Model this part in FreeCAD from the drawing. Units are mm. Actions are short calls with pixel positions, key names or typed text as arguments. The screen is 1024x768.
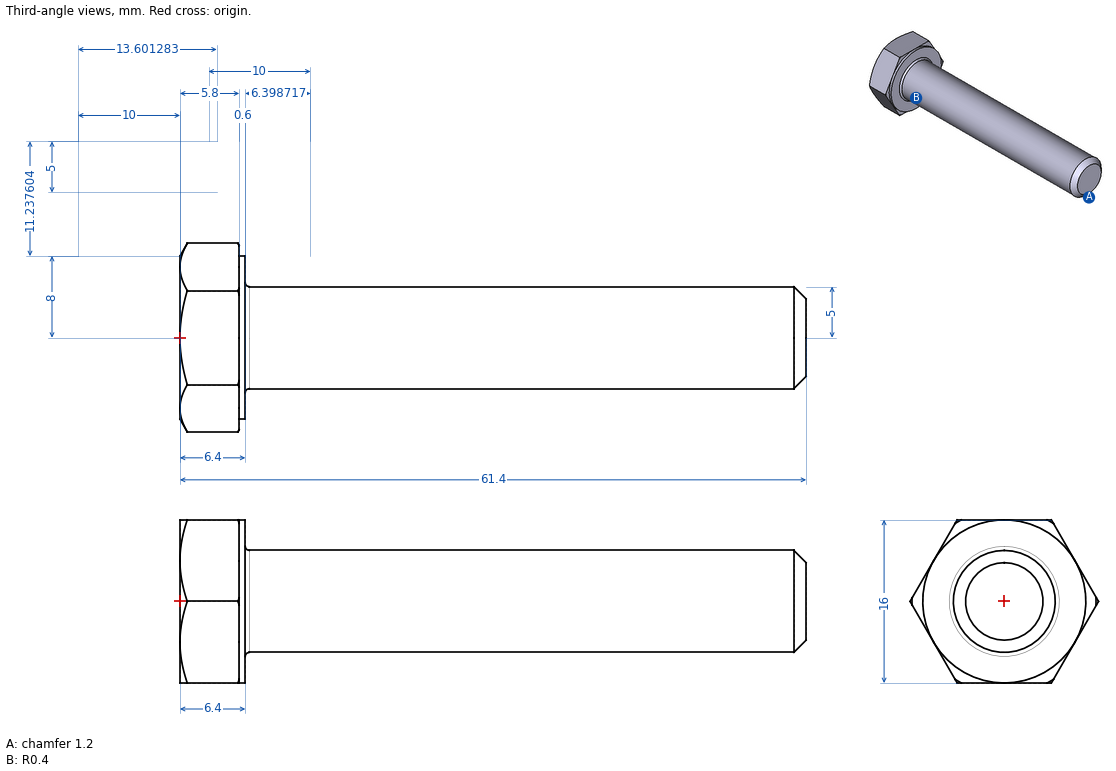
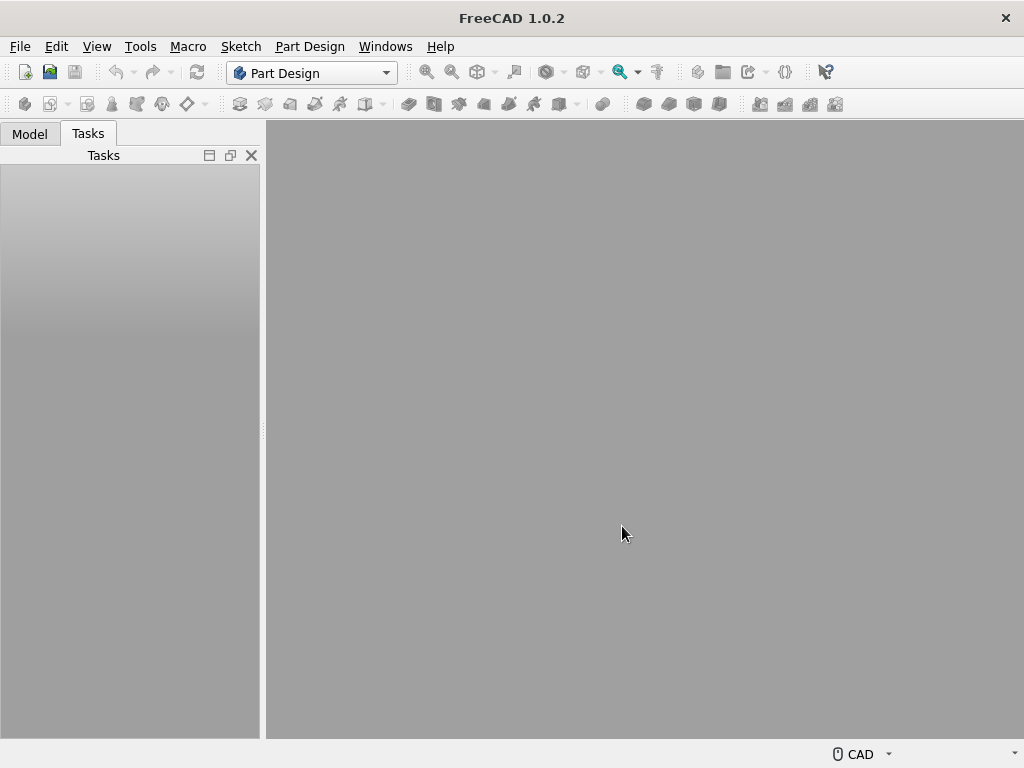
click(25, 72)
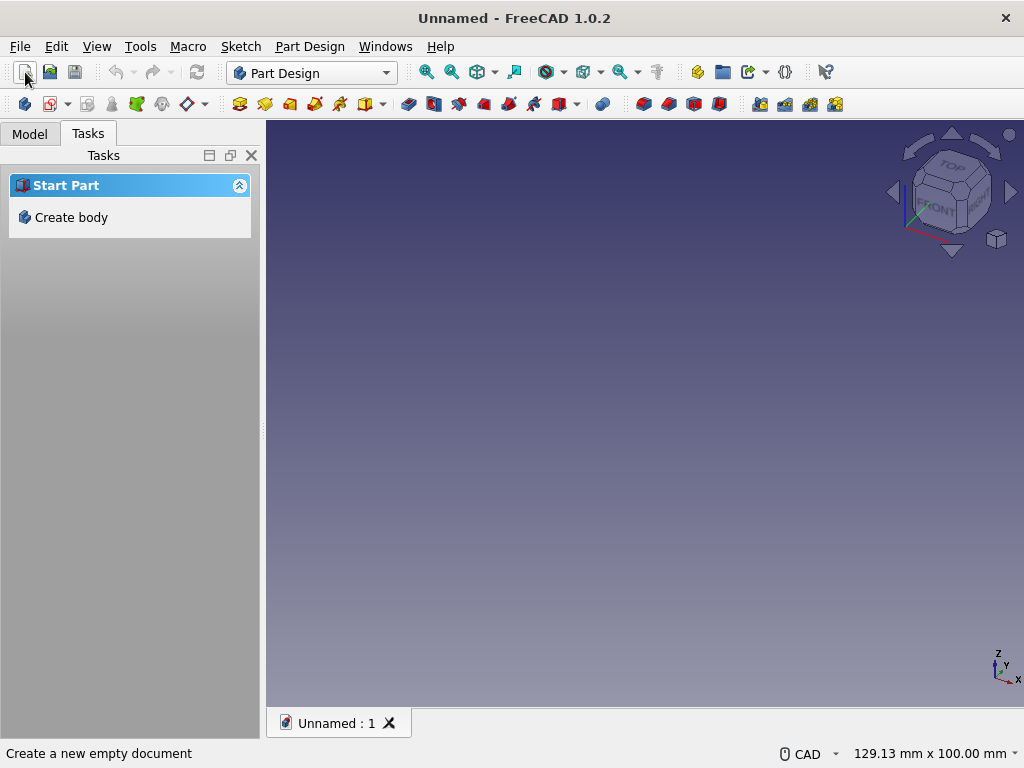
click(50, 104)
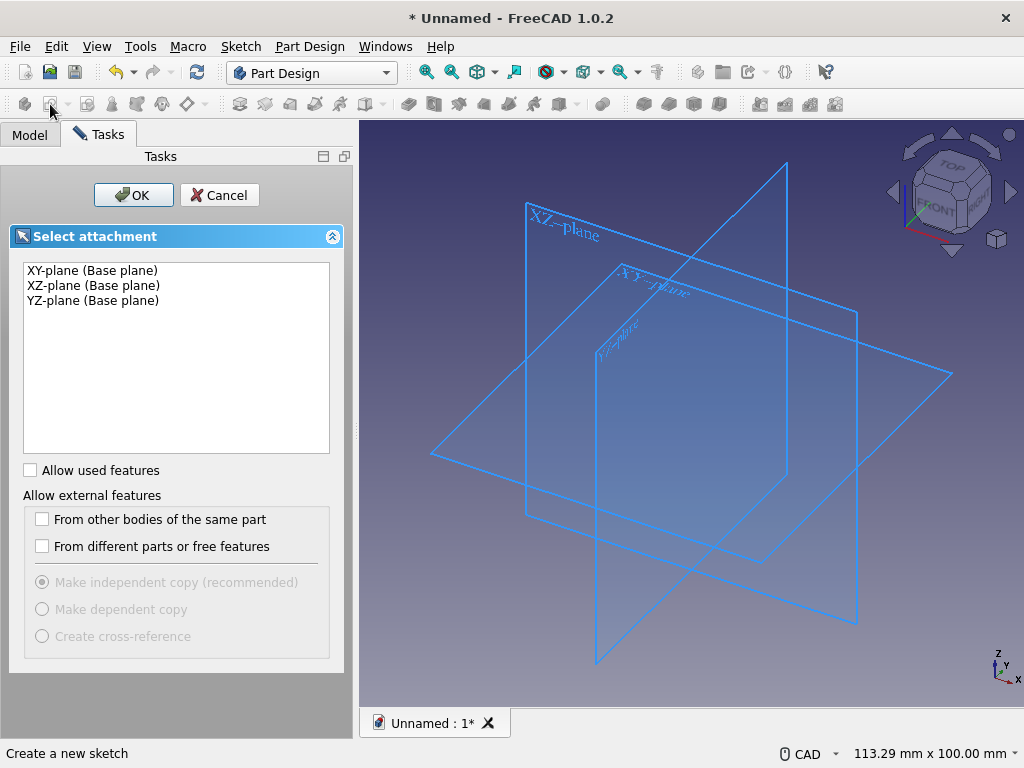
click(84, 300)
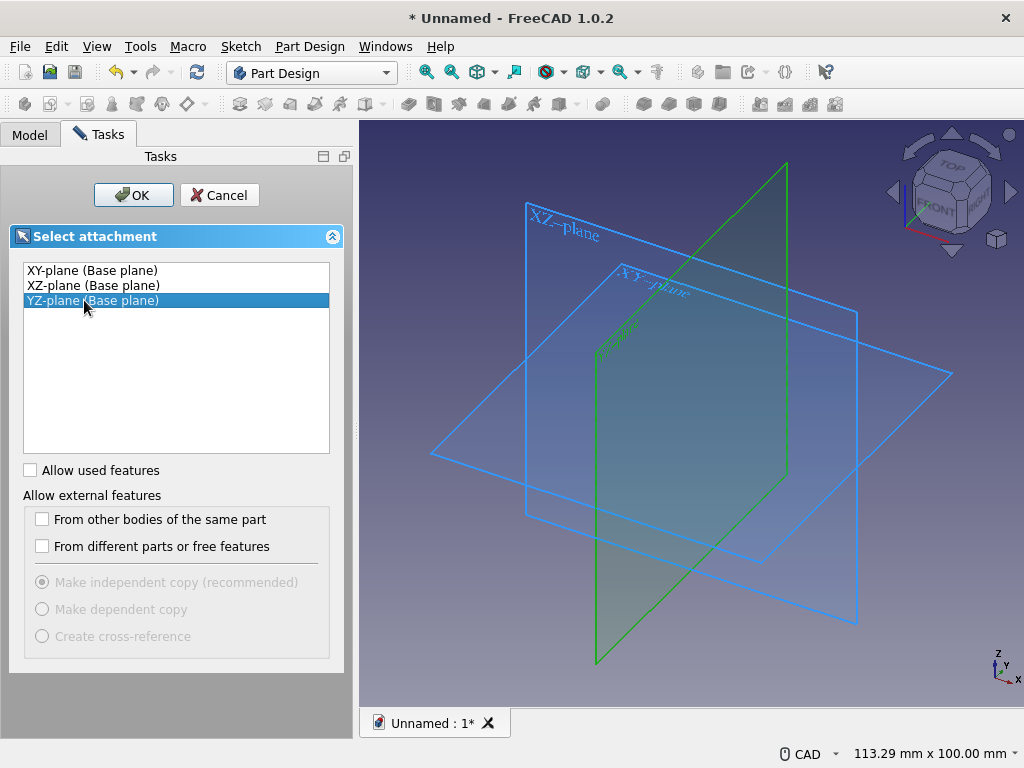
click(134, 195)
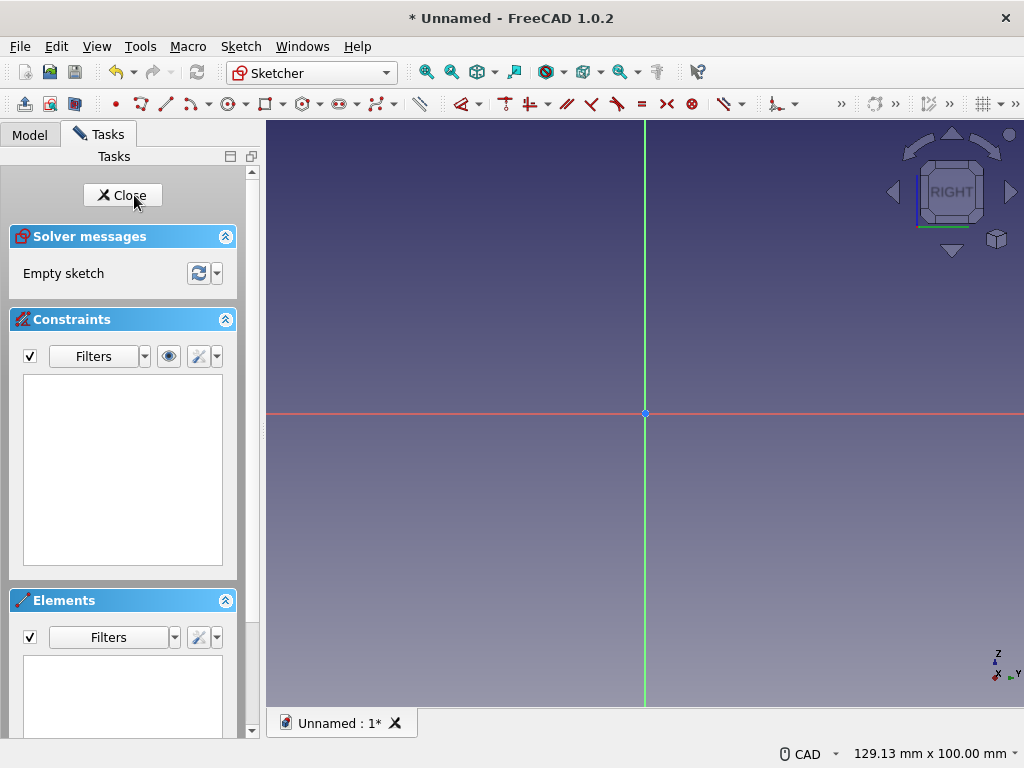
scroll(667, 414, up, 7)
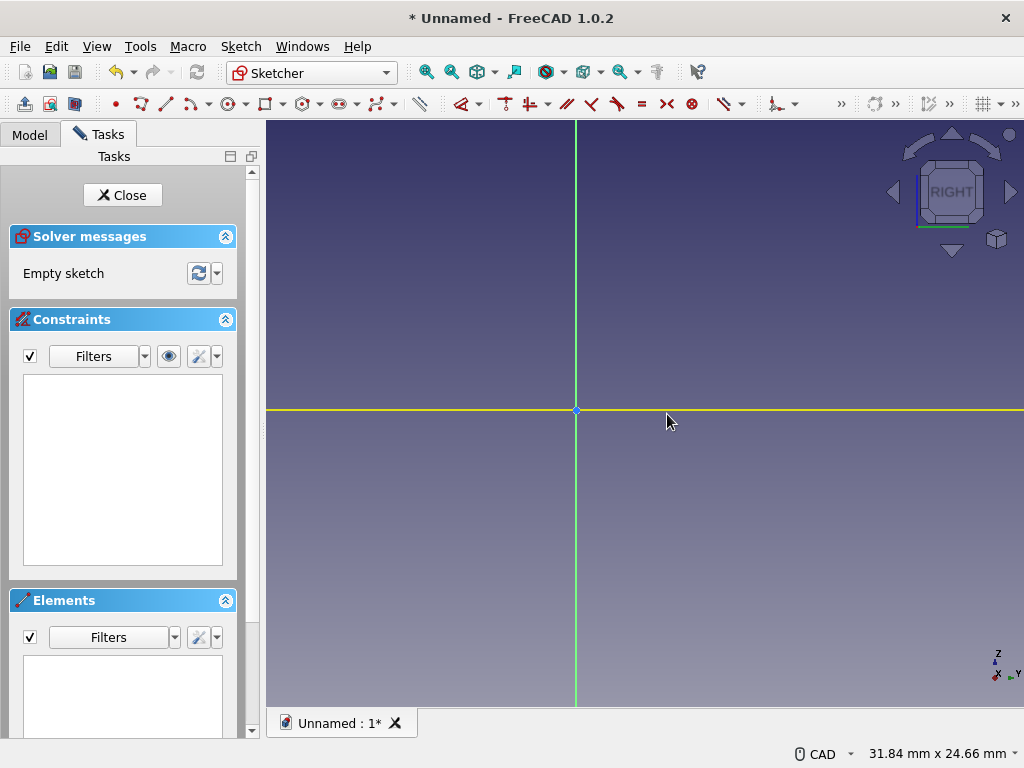
click(302, 104)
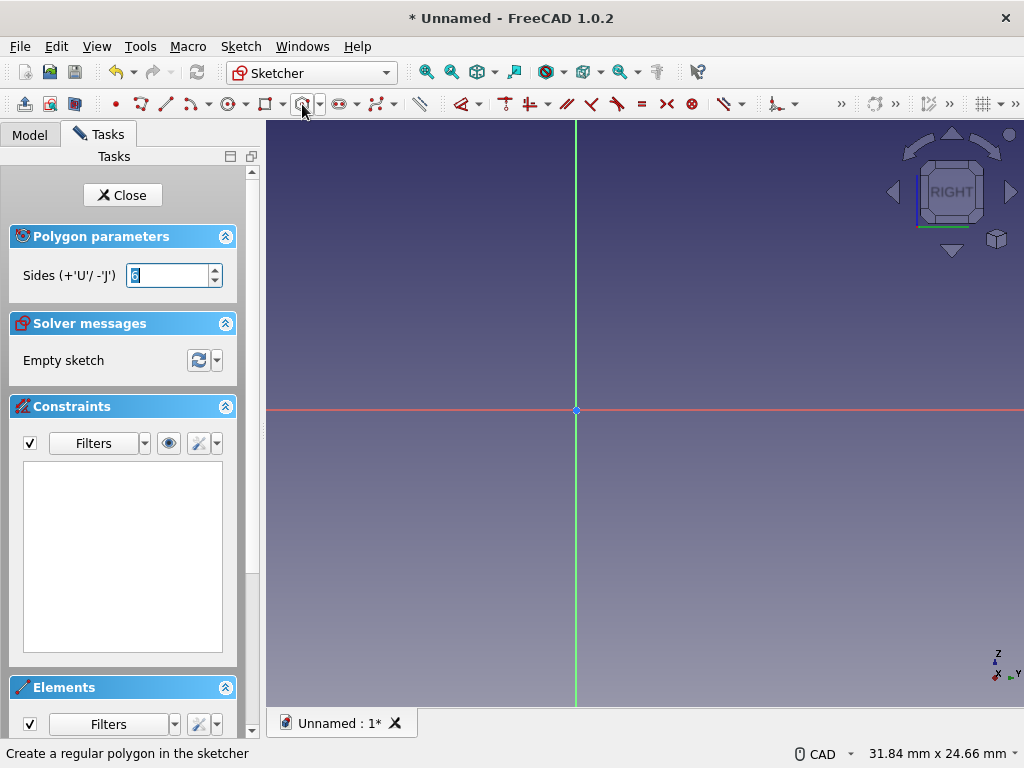
click(576, 410)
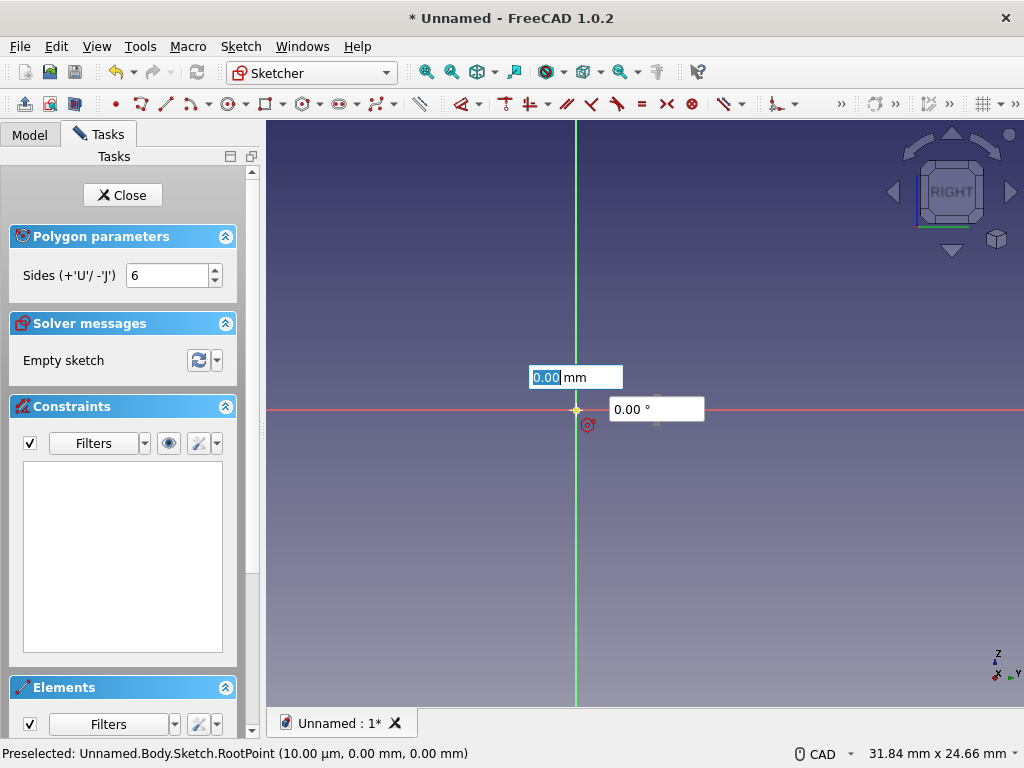
click(796, 410)
right_click(796, 410)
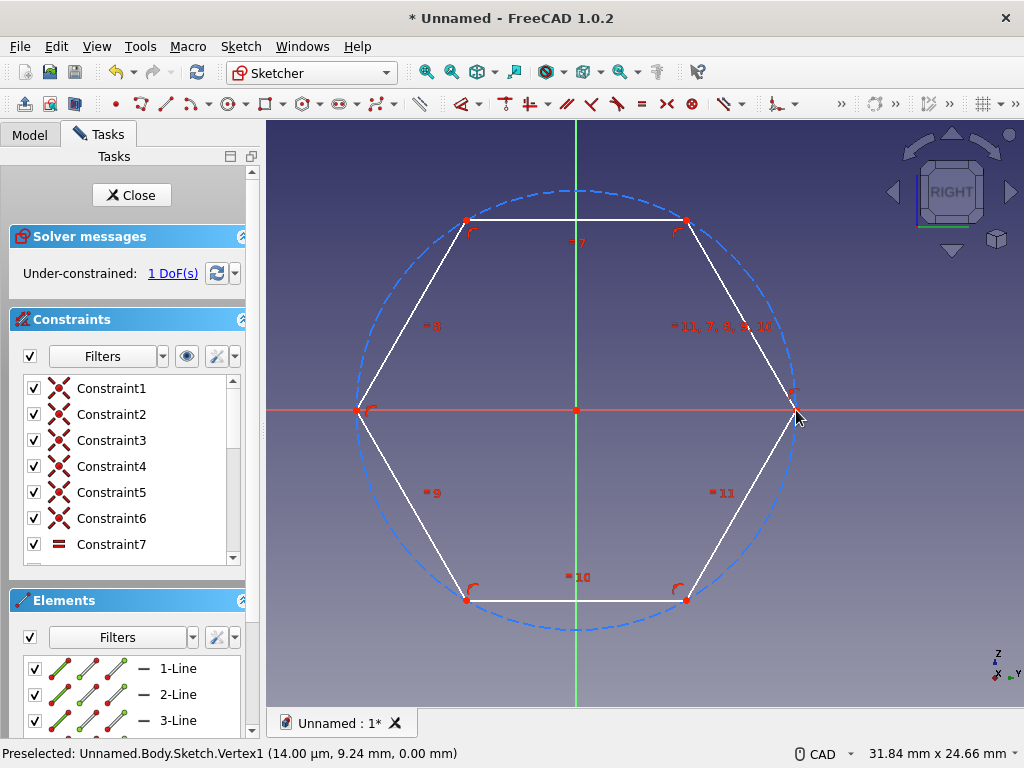
click(466, 601)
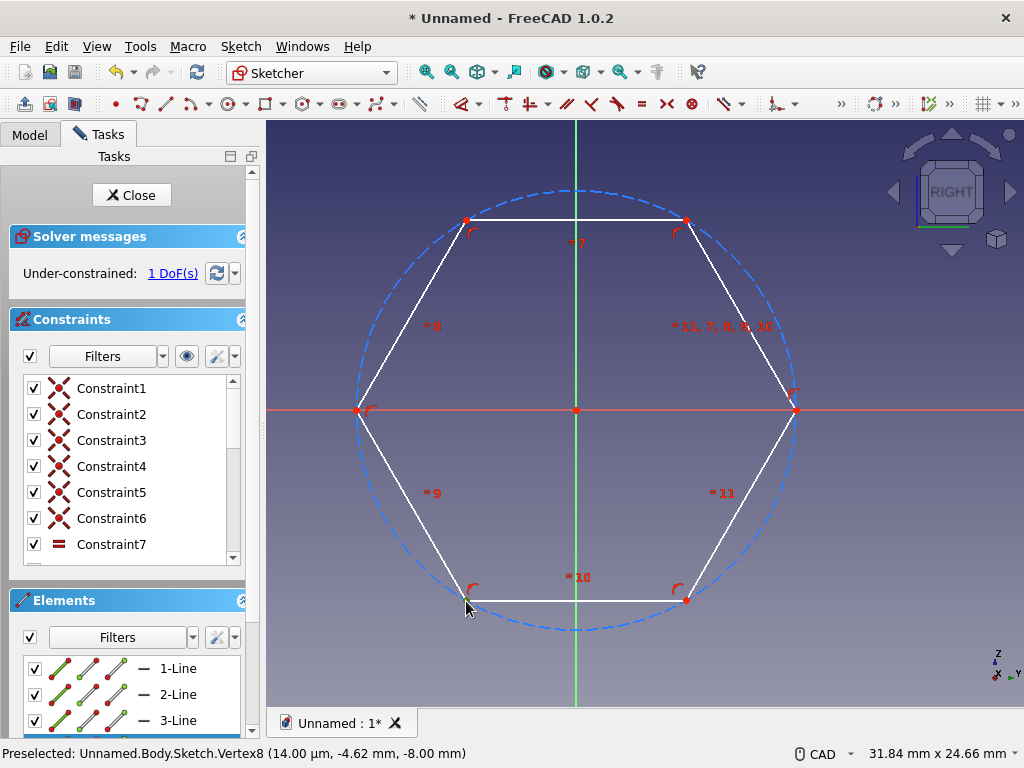
click(686, 220)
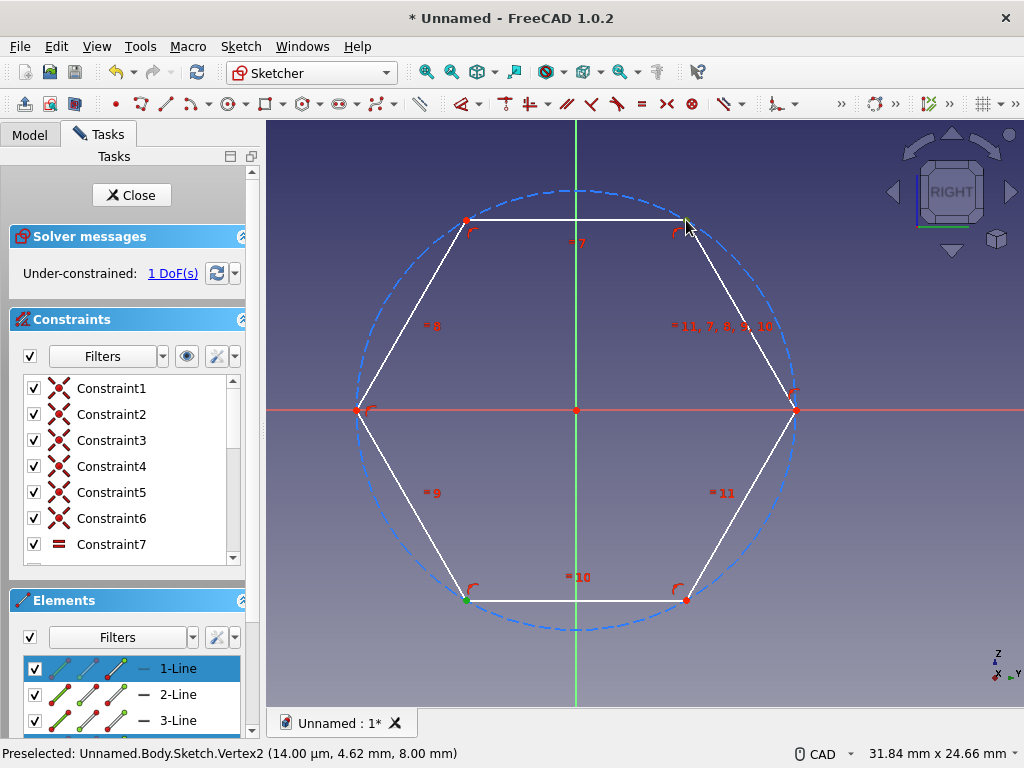
key(i)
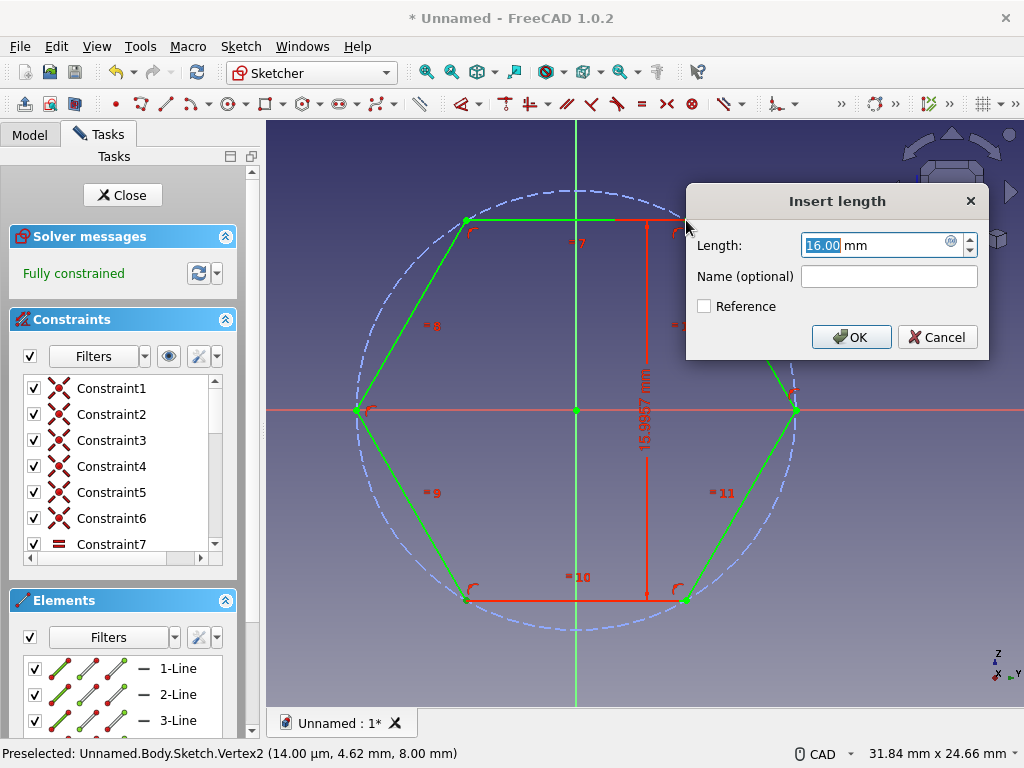
text(16)
key(Return)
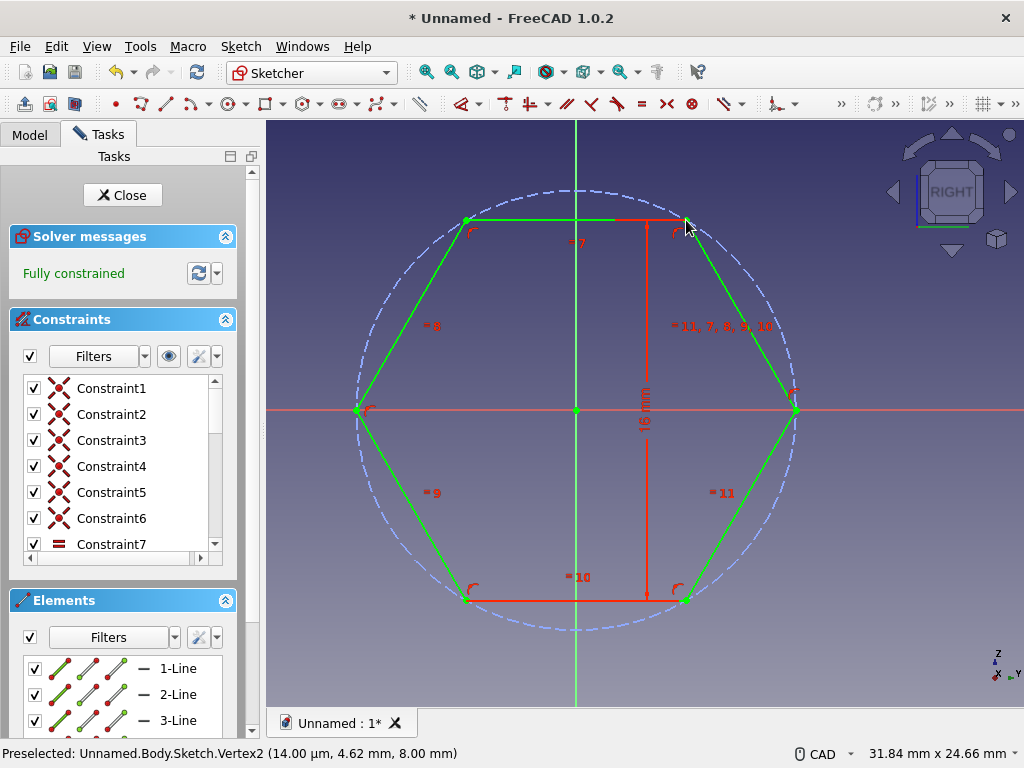
click(123, 195)